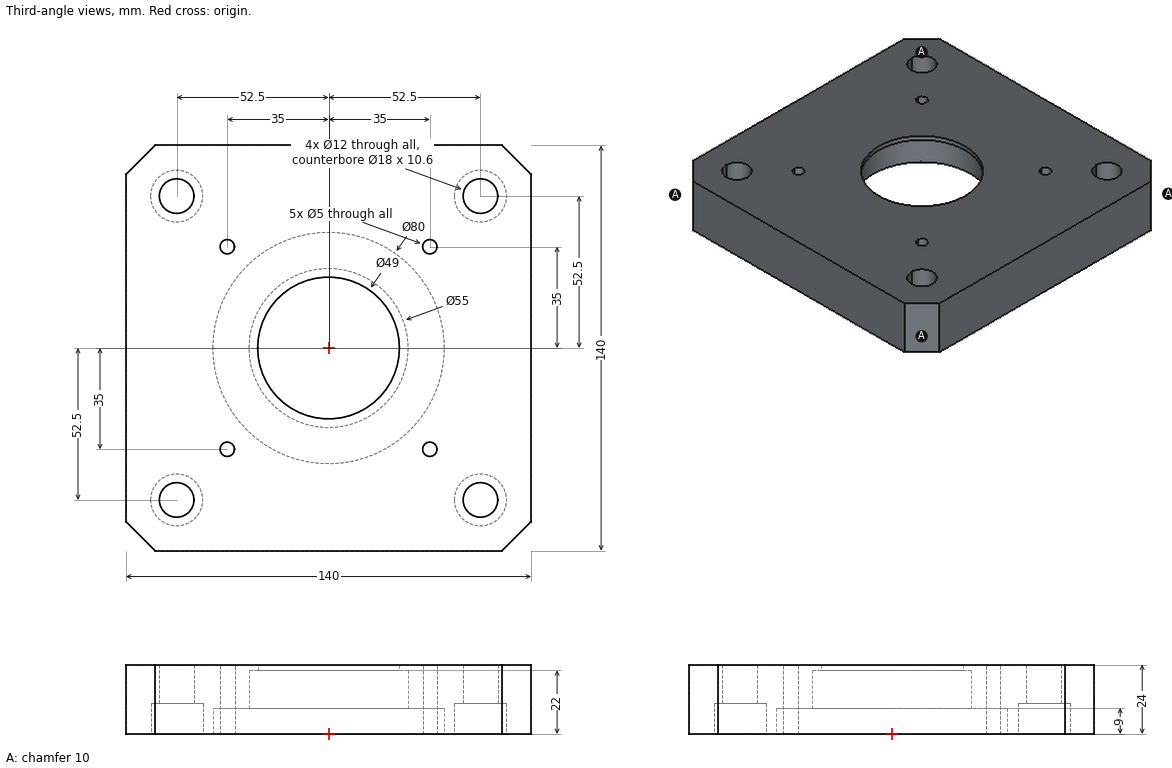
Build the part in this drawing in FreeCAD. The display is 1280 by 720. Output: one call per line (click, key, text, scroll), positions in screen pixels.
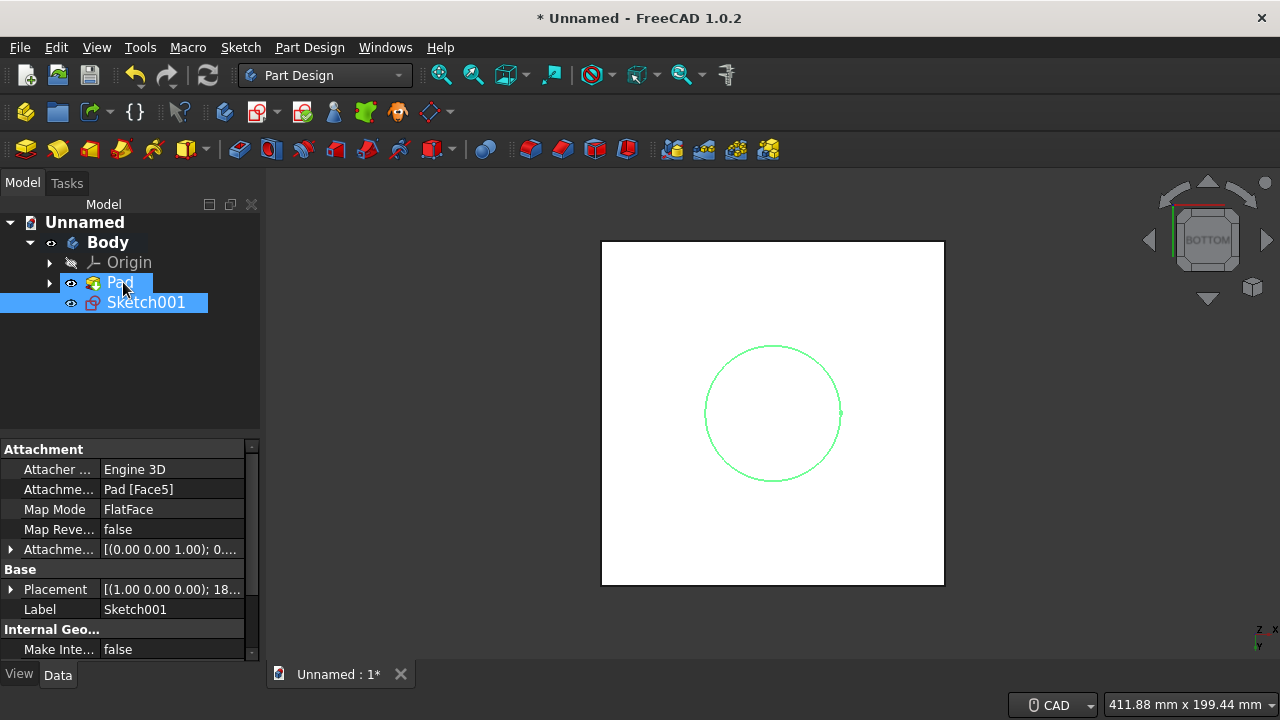
click(240, 150)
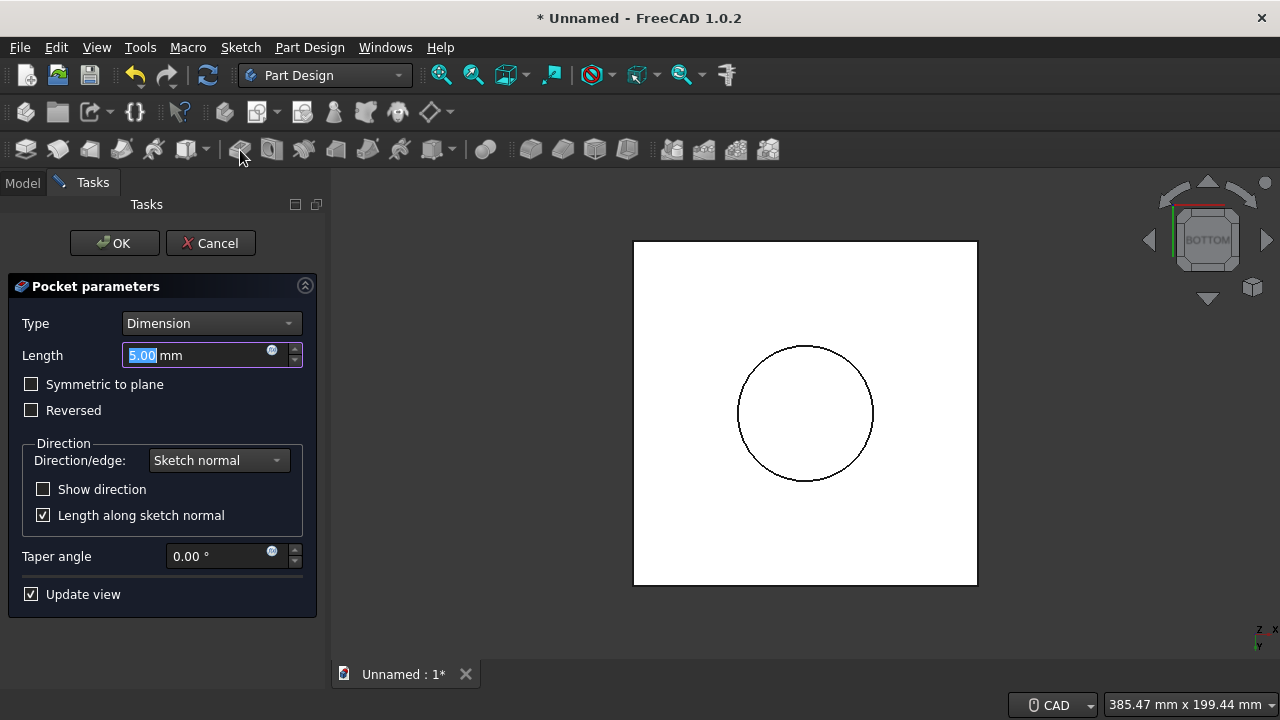
text(22)
key(Tab)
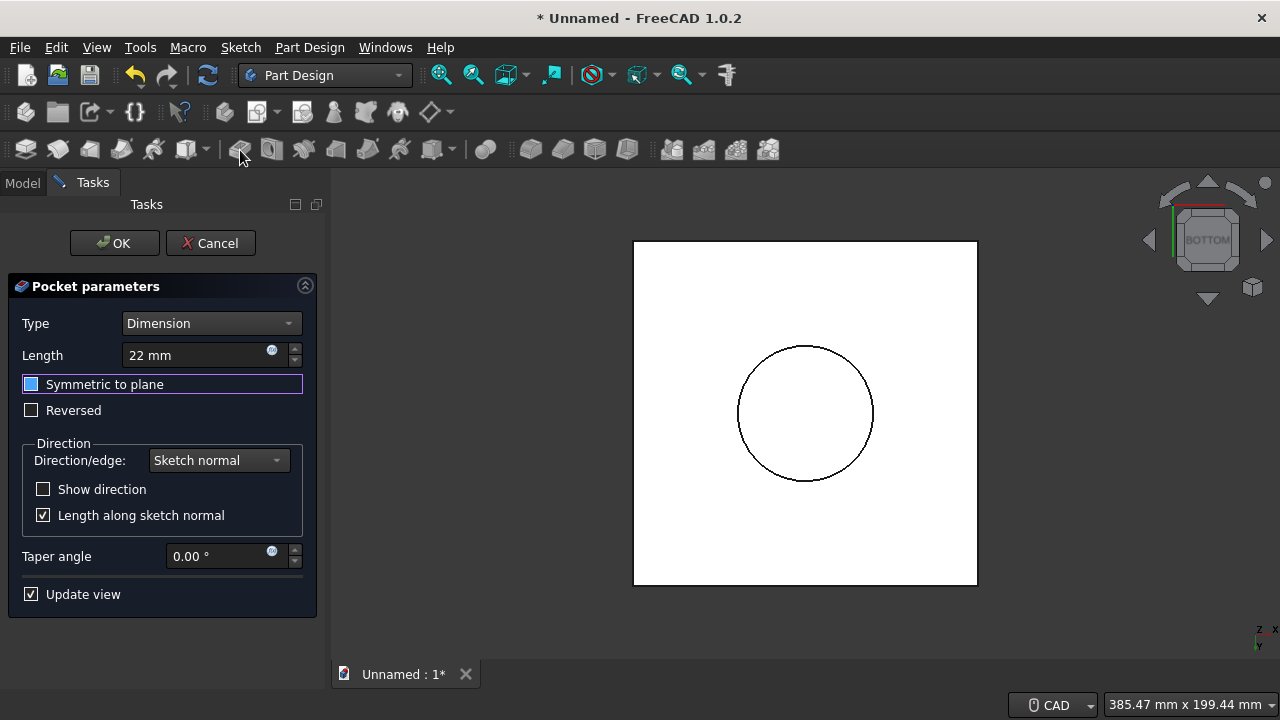
click(115, 243)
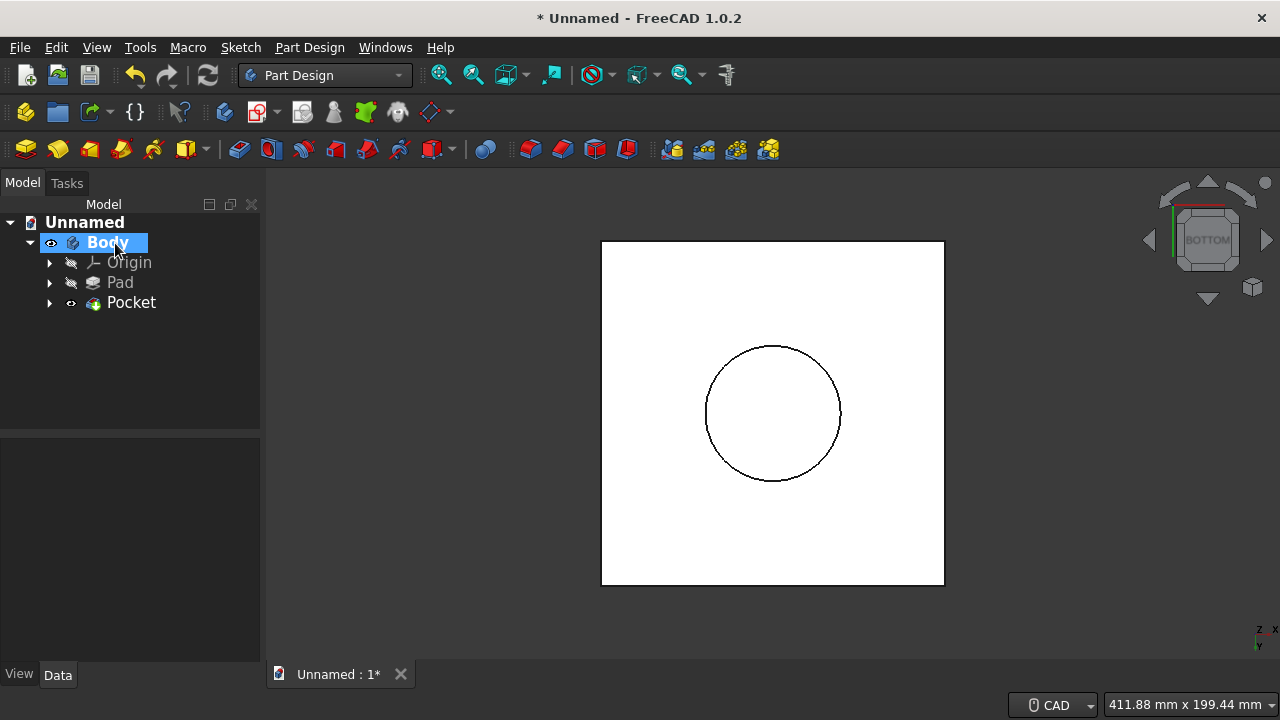
click(773, 413)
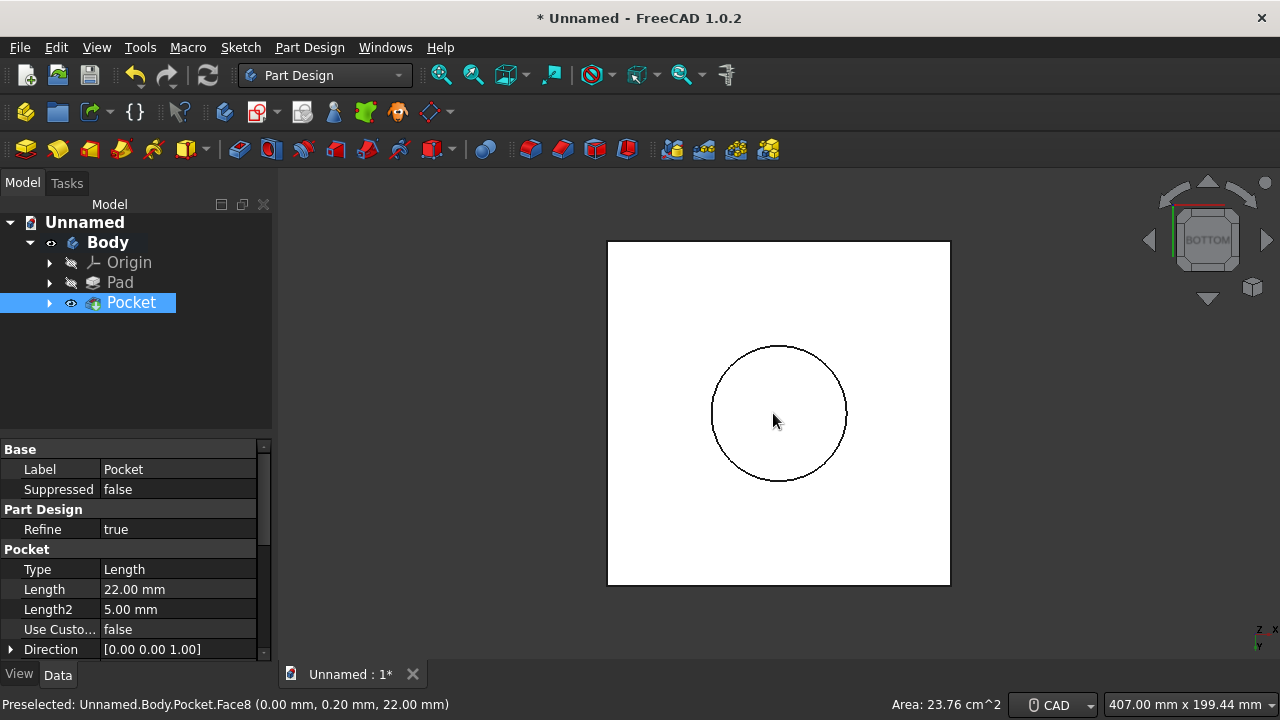
click(258, 112)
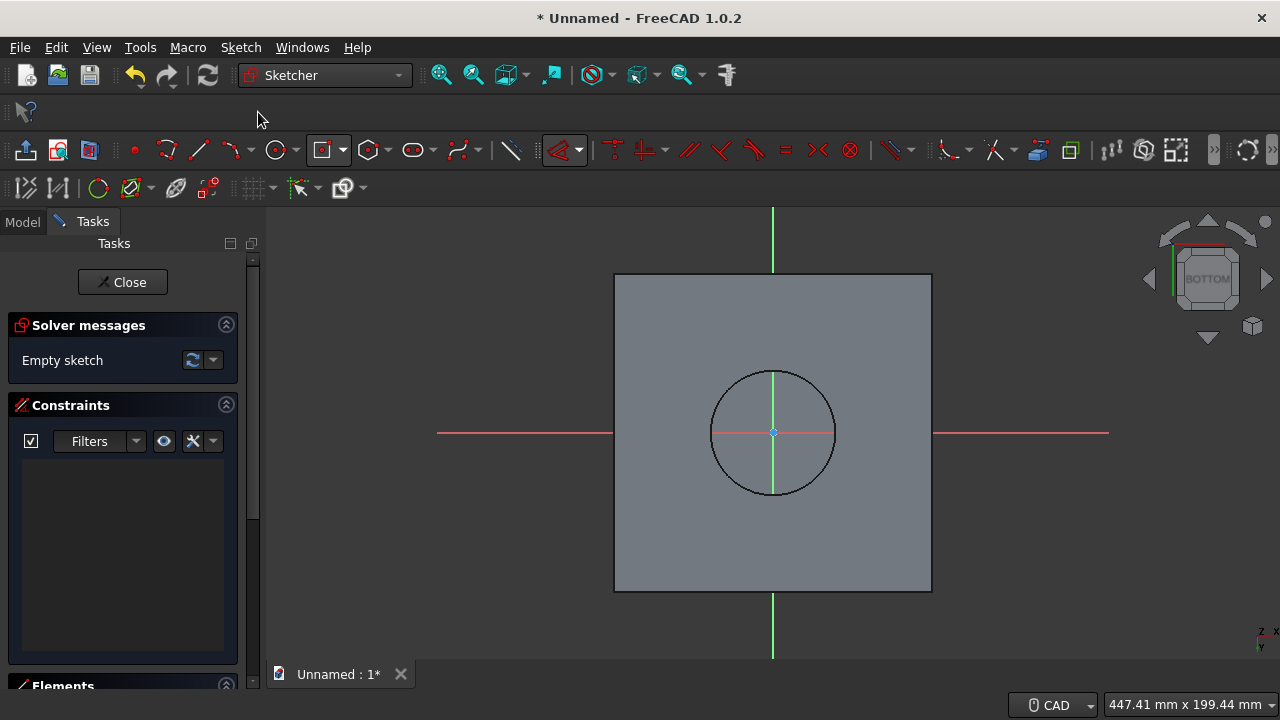
click(90, 150)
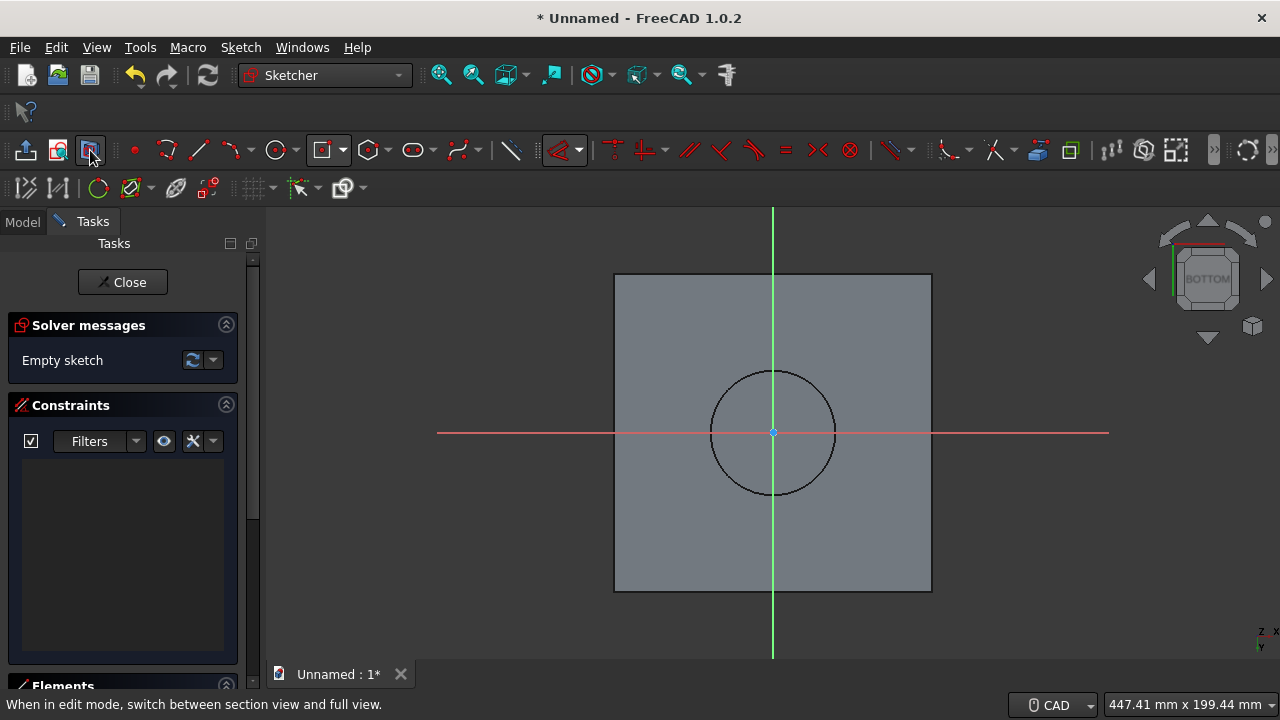
scroll(813, 433, up, 5)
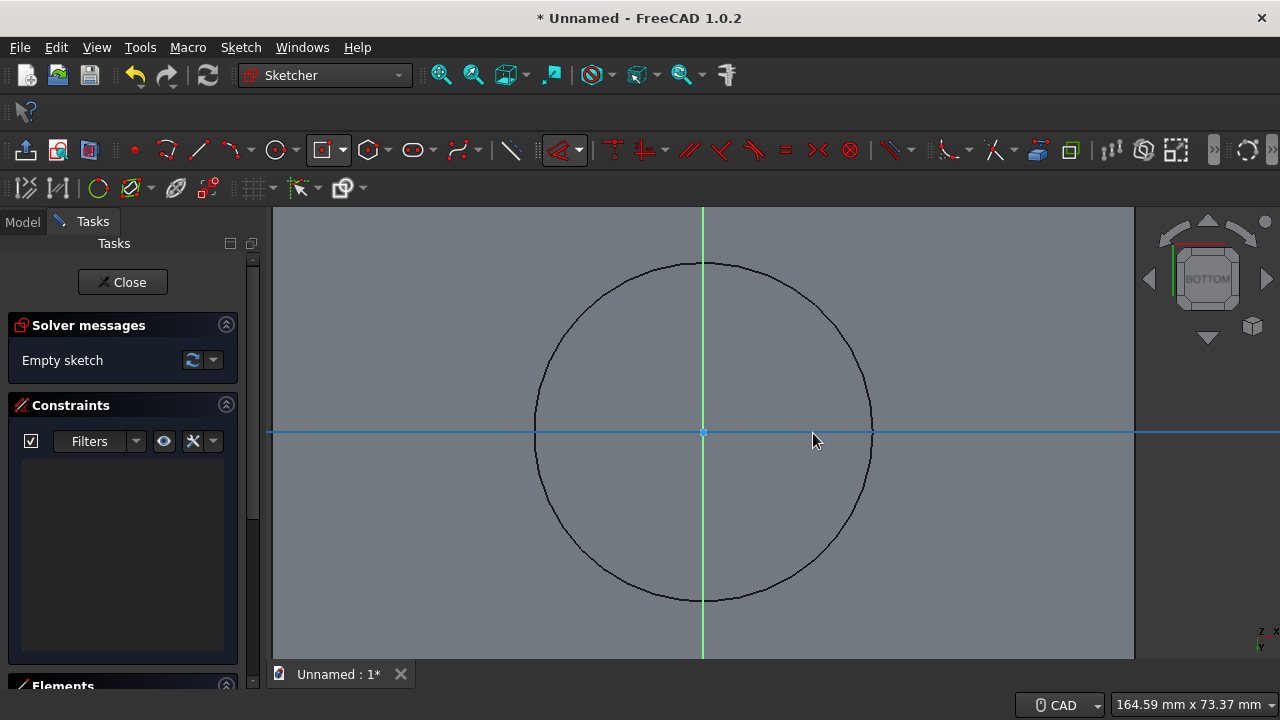
click(276, 150)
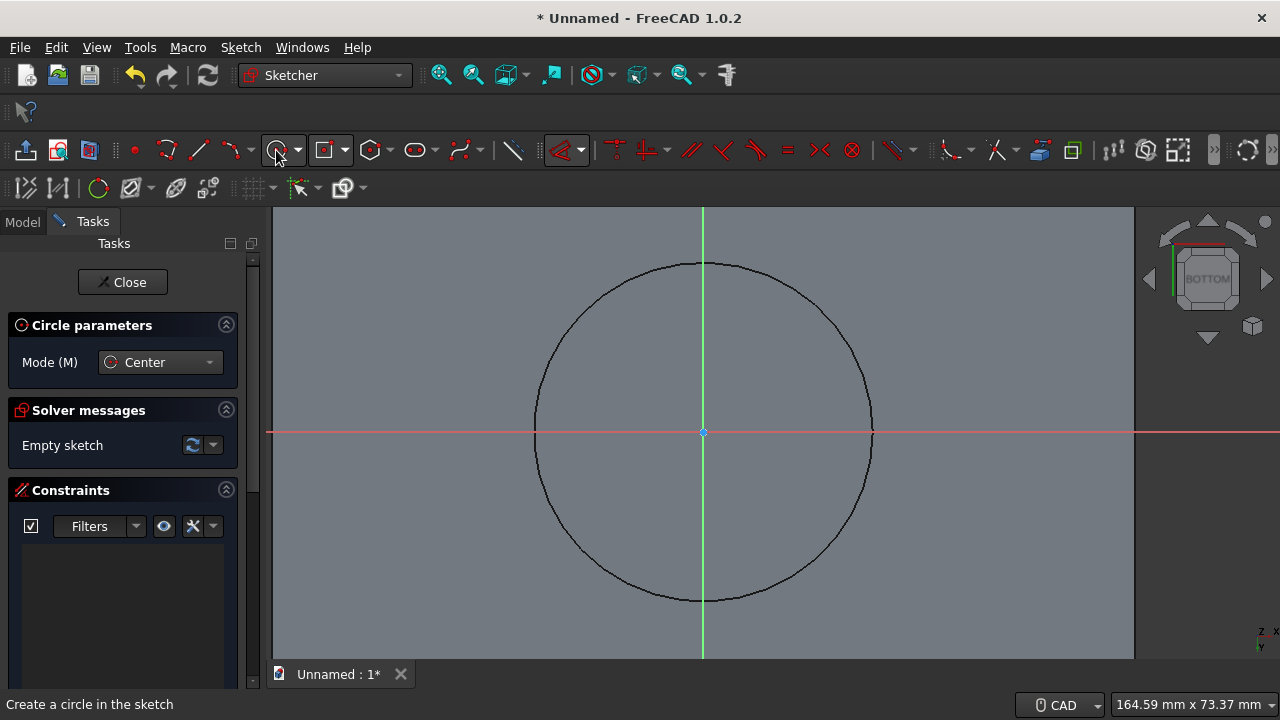
click(703, 432)
move(810, 325)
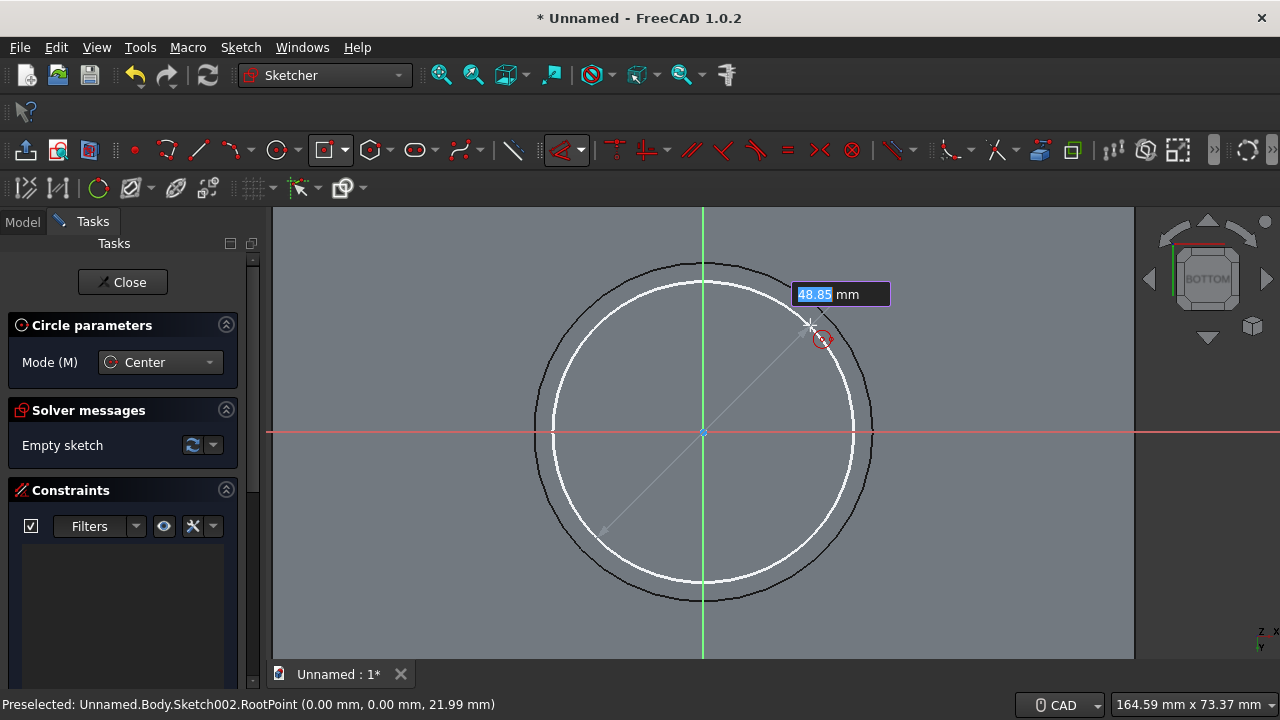
text(49)
key(Return)
key(Escape)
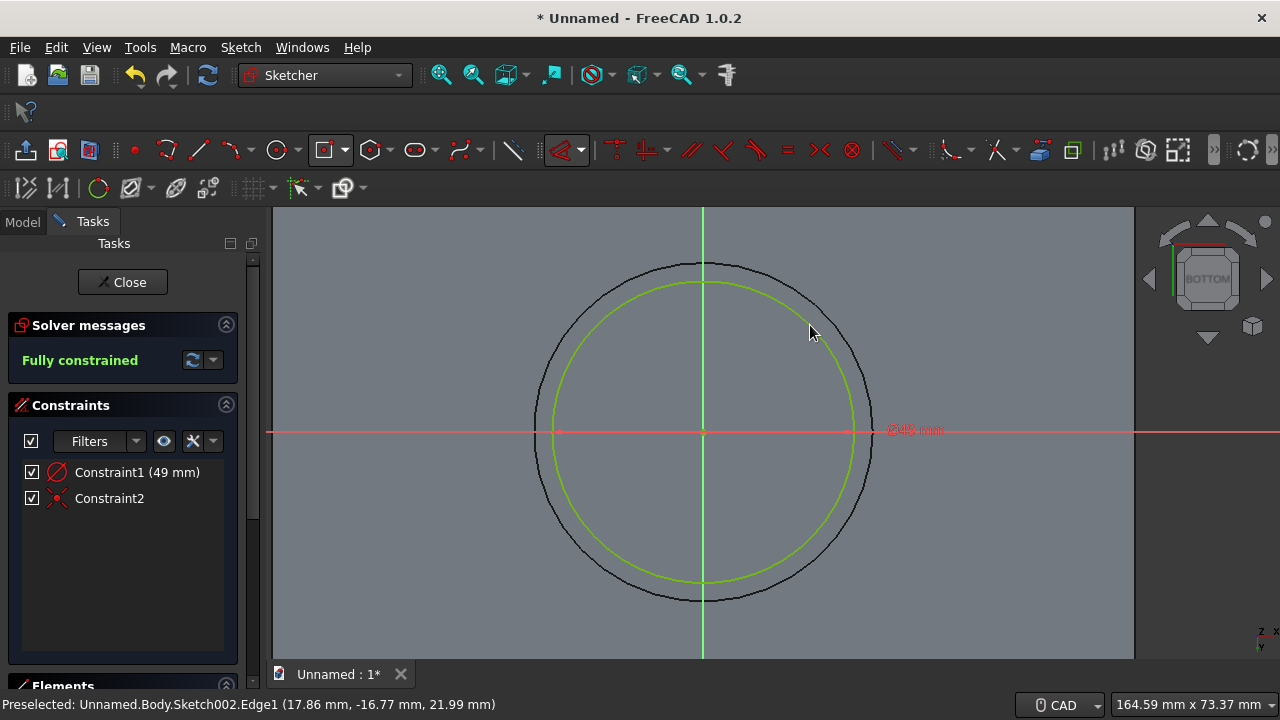
click(123, 282)